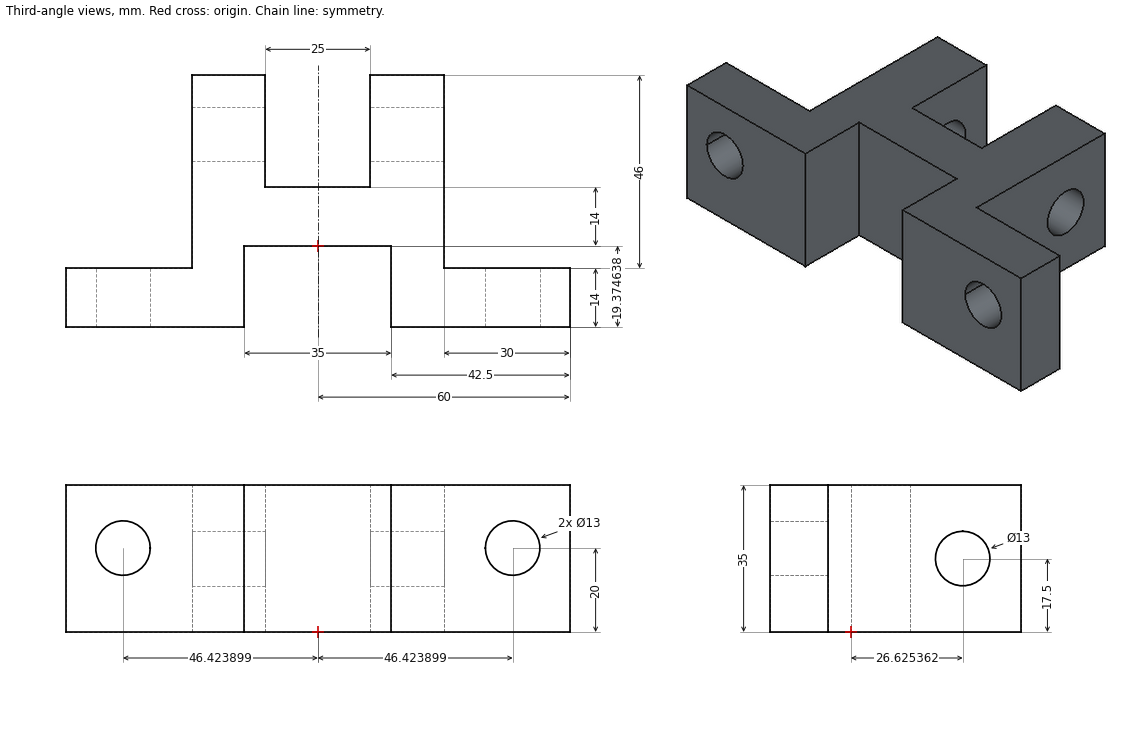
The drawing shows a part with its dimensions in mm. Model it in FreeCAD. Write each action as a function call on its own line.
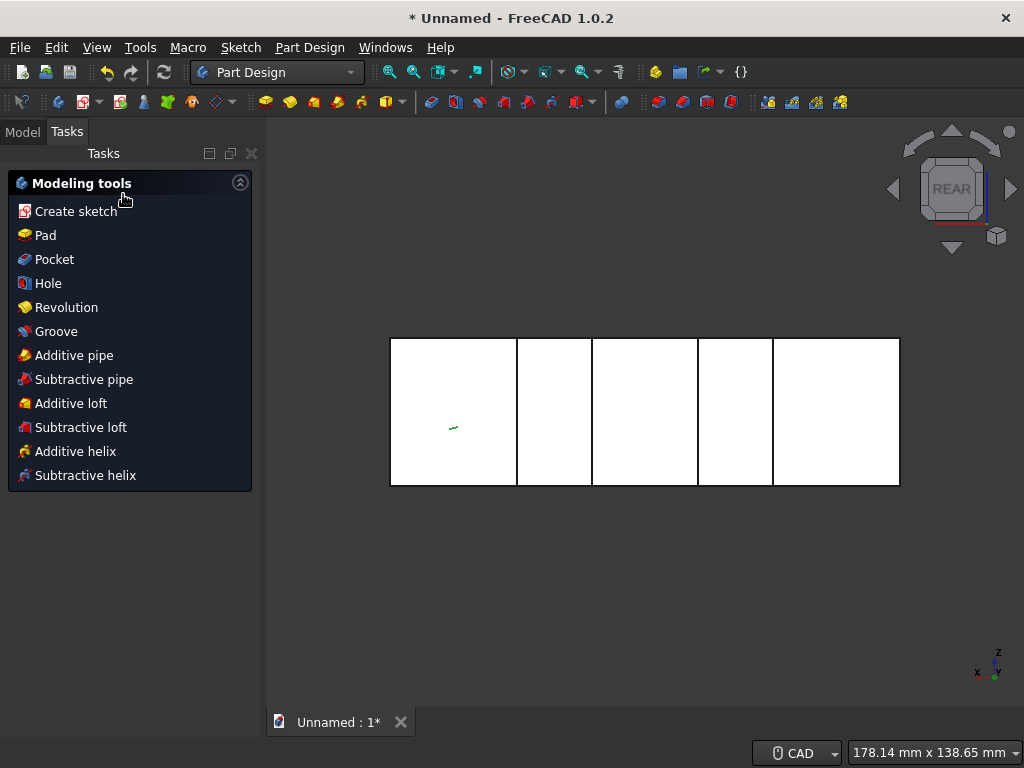
click(432, 102)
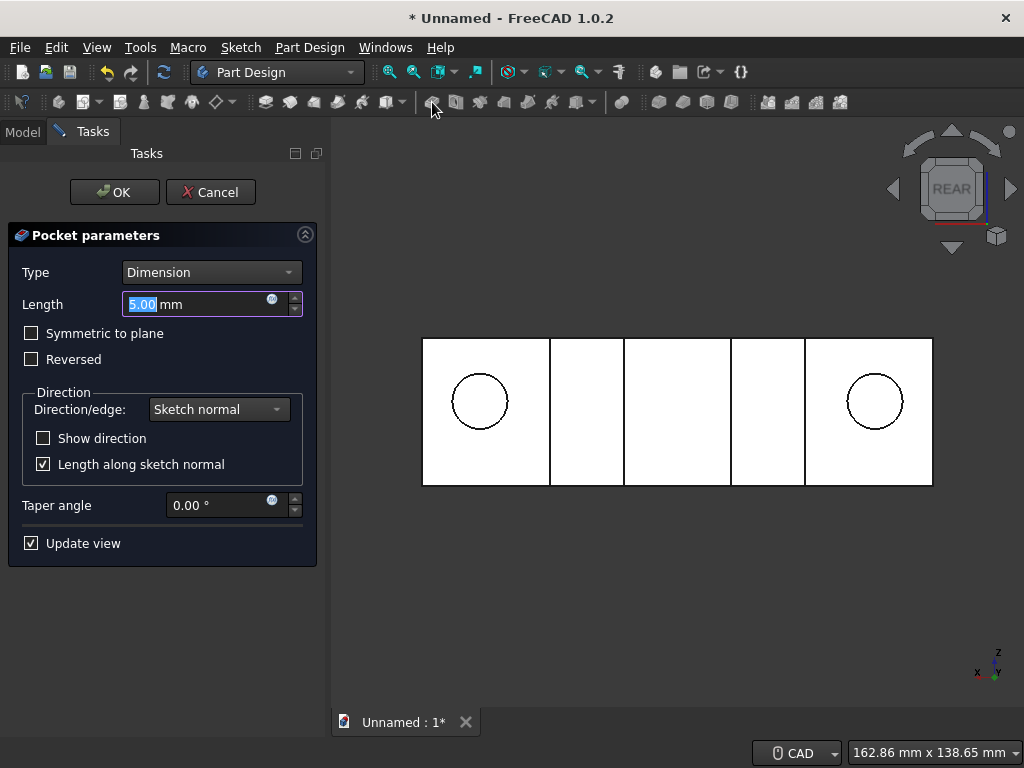
click(212, 272)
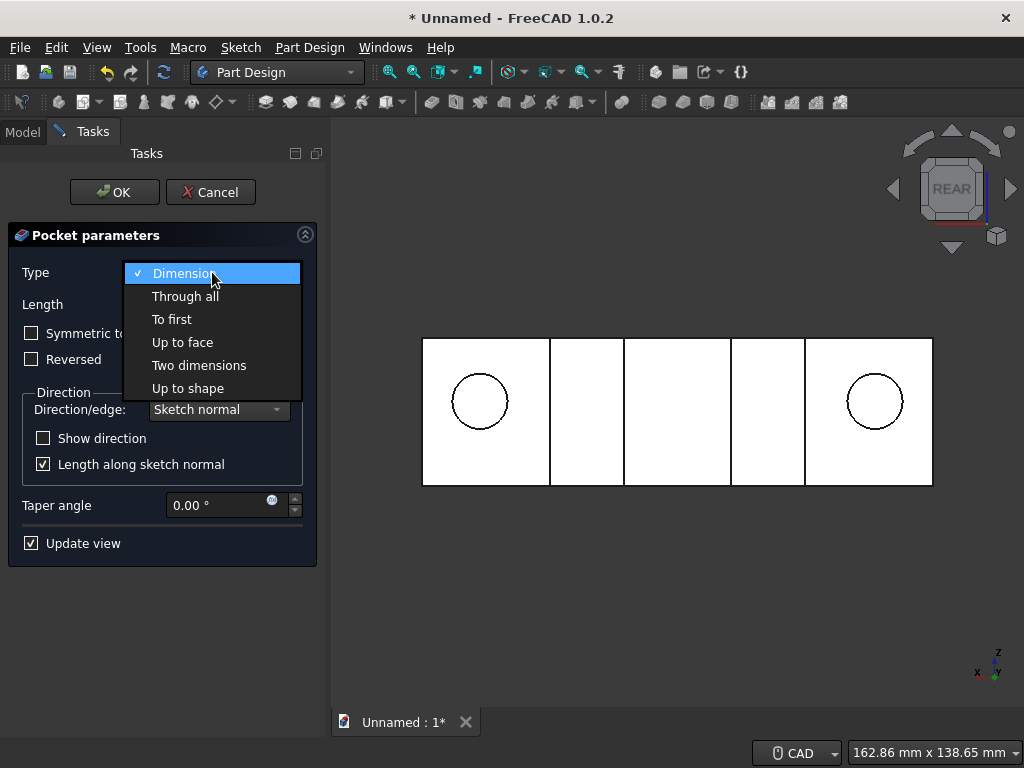
click(212, 296)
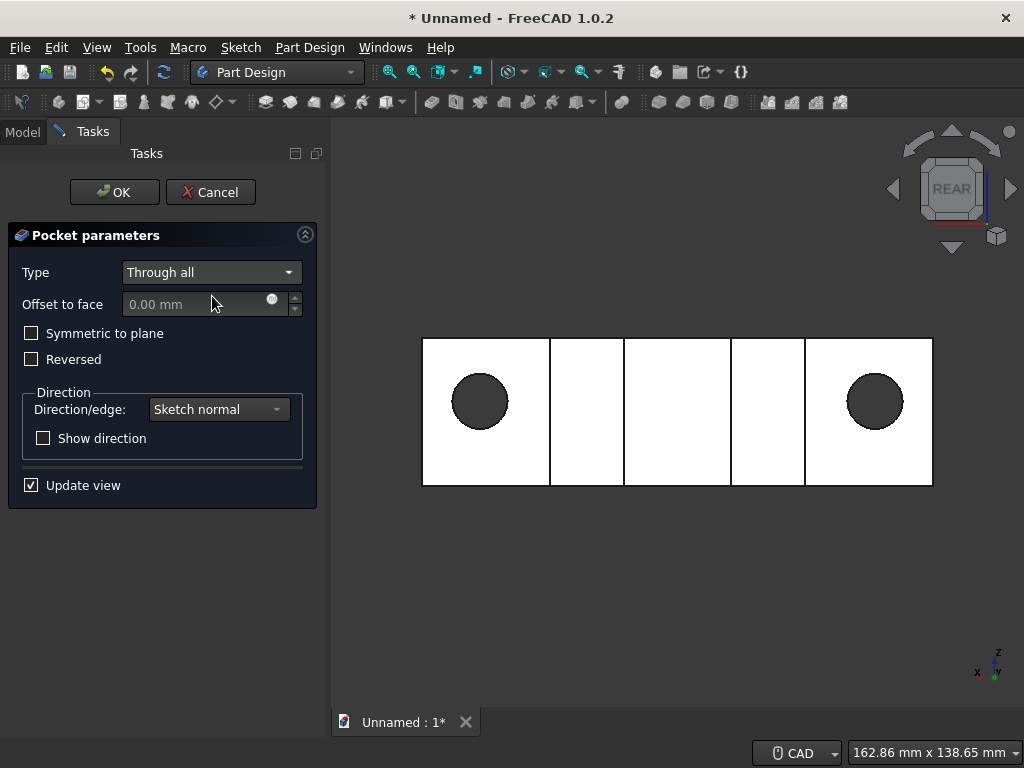
click(115, 192)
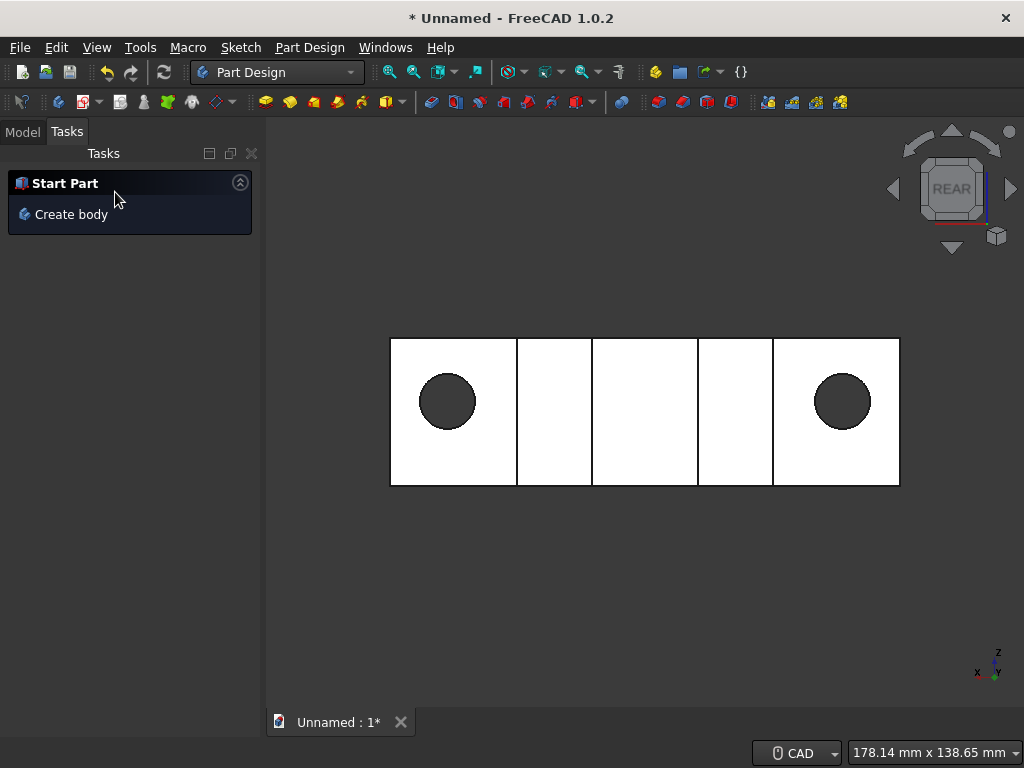
key(0)